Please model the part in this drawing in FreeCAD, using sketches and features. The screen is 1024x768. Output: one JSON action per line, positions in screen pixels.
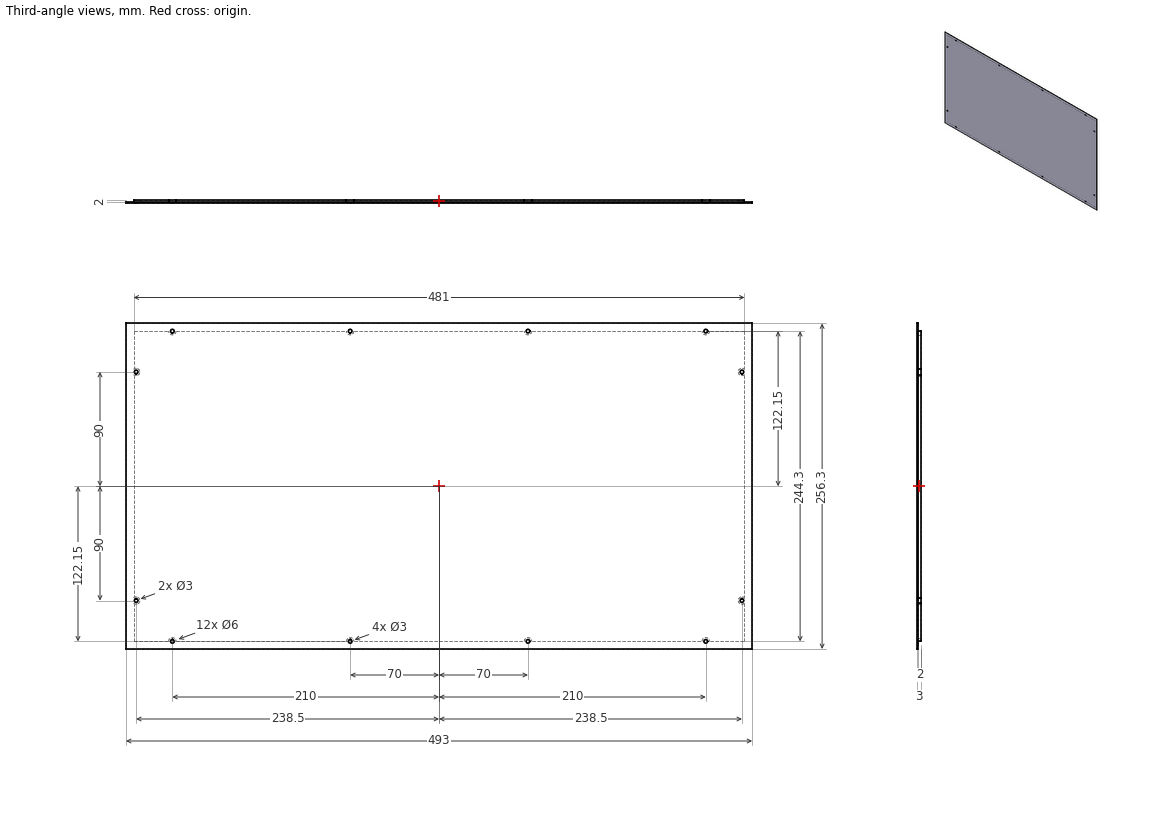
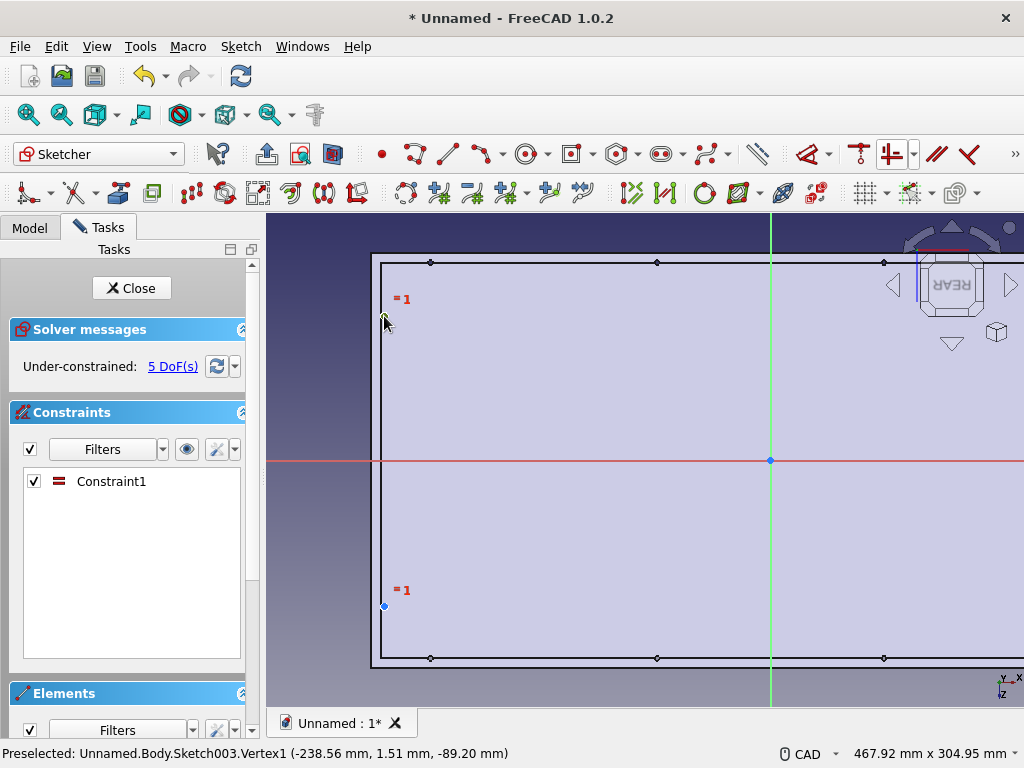
{"action": "left_click", "coordinate": [384, 607]}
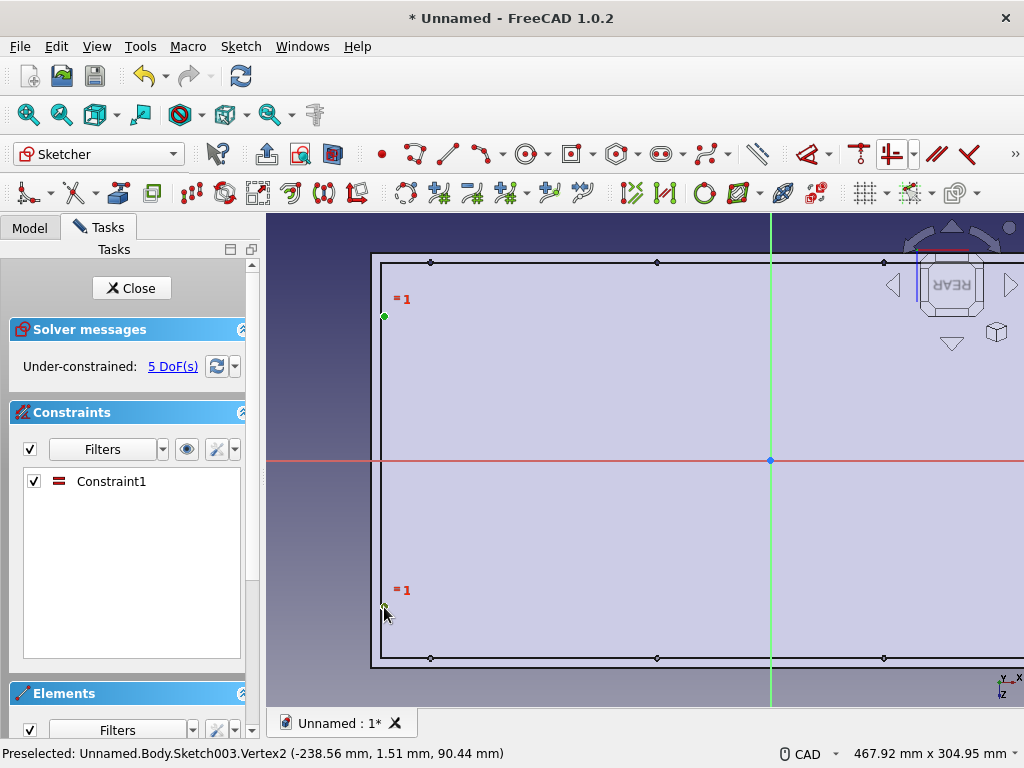
{"action": "key", "text": "v"}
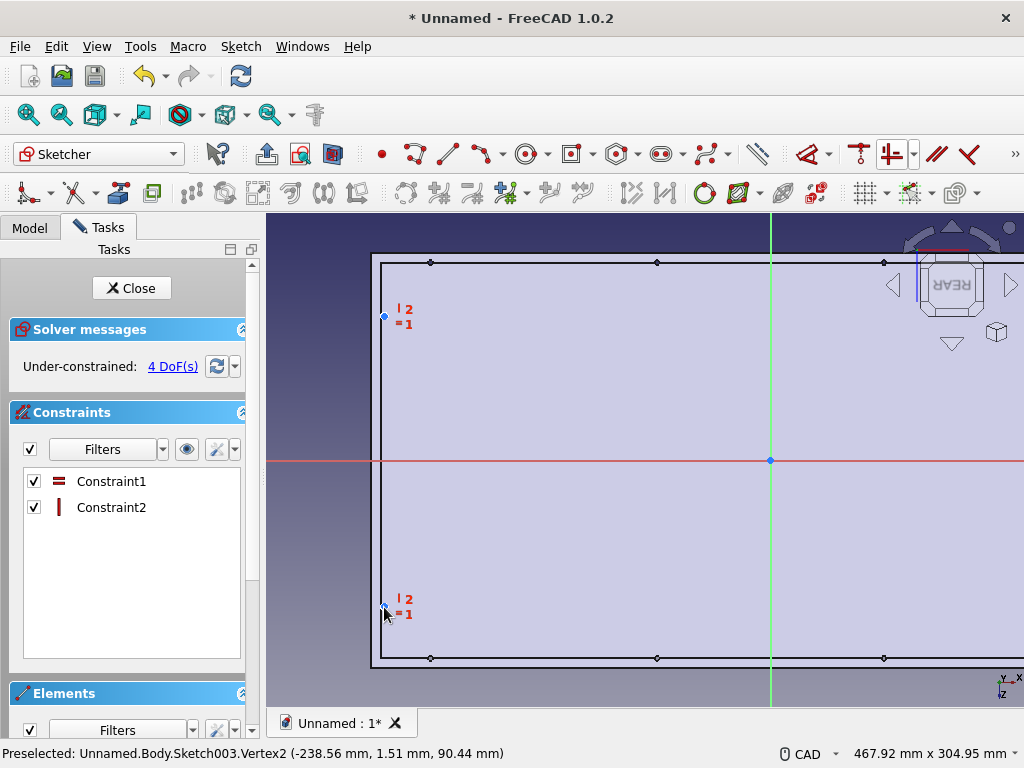
{"action": "left_click", "coordinate": [806, 154]}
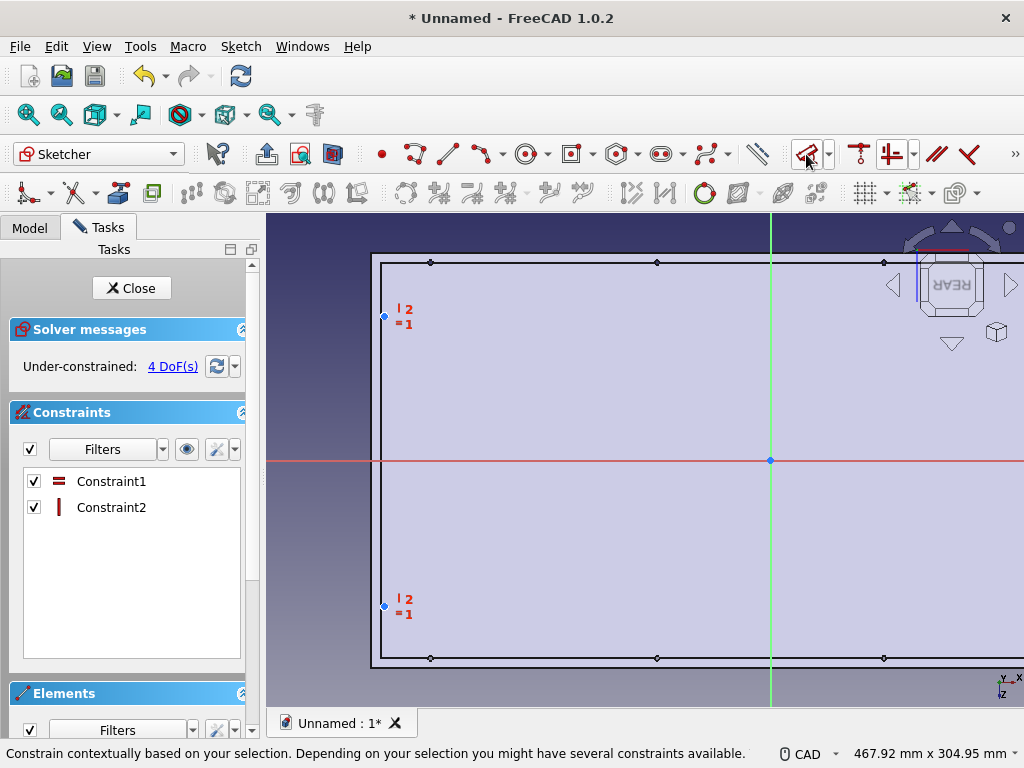
{"action": "scroll", "coordinate": [381, 316], "scroll_direction": "up", "scroll_amount": 11}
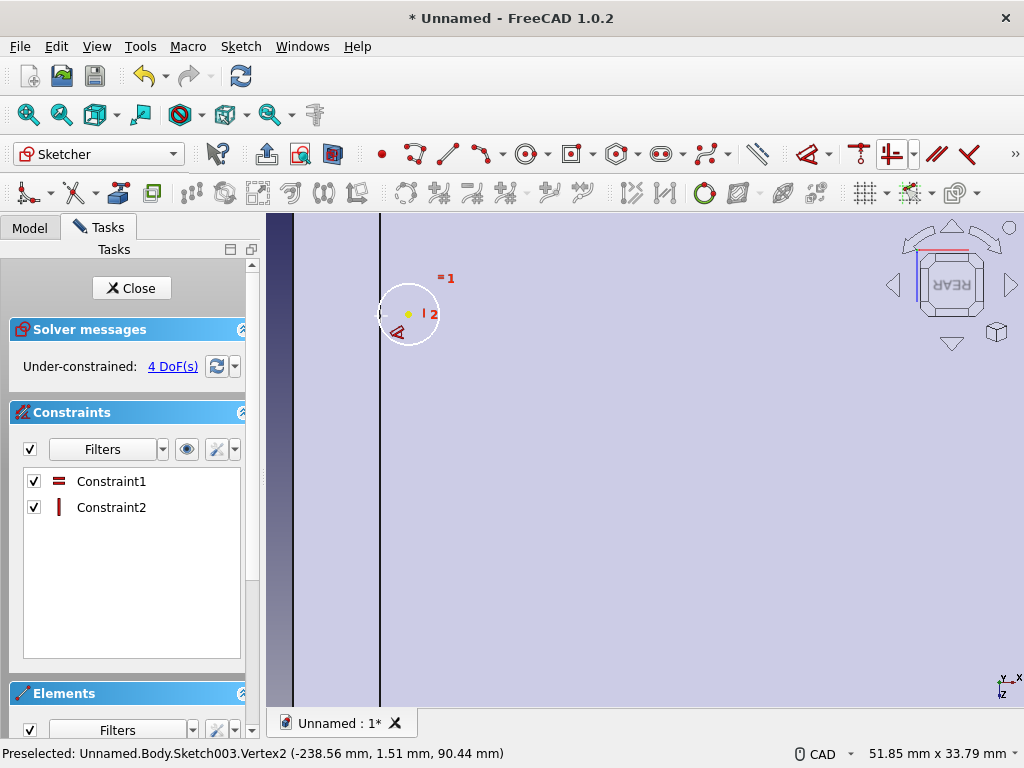
{"action": "left_click", "coordinate": [378, 313]}
{"action": "left_click", "coordinate": [346, 312]}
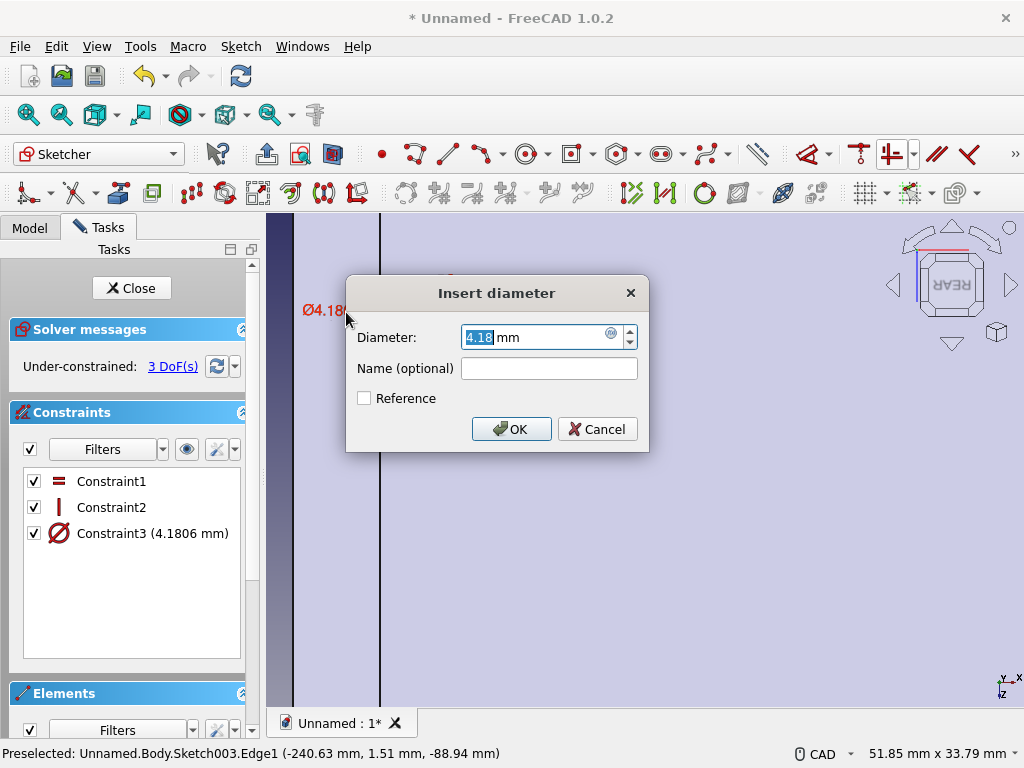
{"action": "type", "text": "3"}
{"action": "key", "text": "Return"}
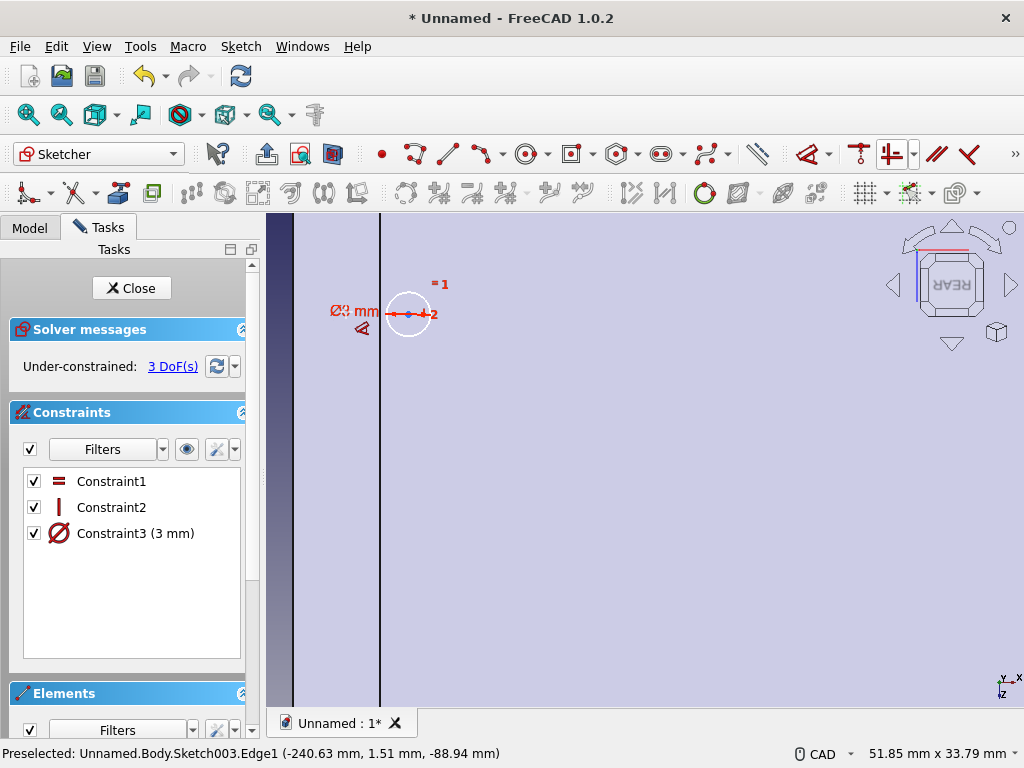
{"action": "scroll", "coordinate": [381, 316], "scroll_direction": "down", "scroll_amount": 11}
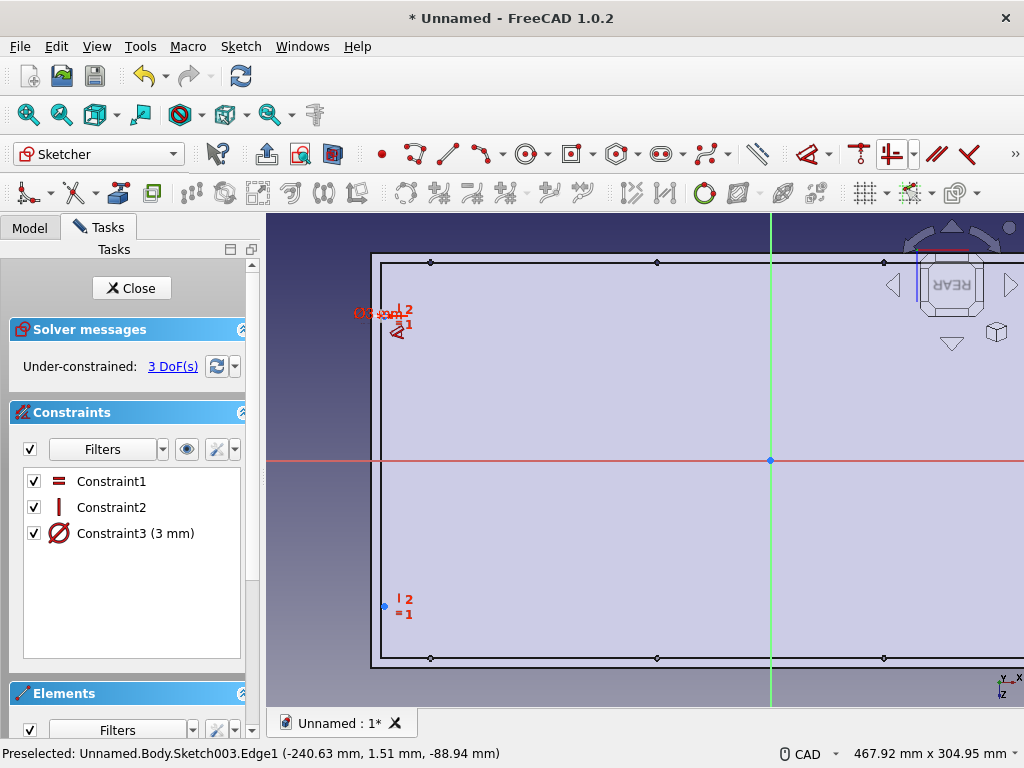
{"action": "left_click", "coordinate": [384, 316]}
{"action": "left_click", "coordinate": [805, 388]}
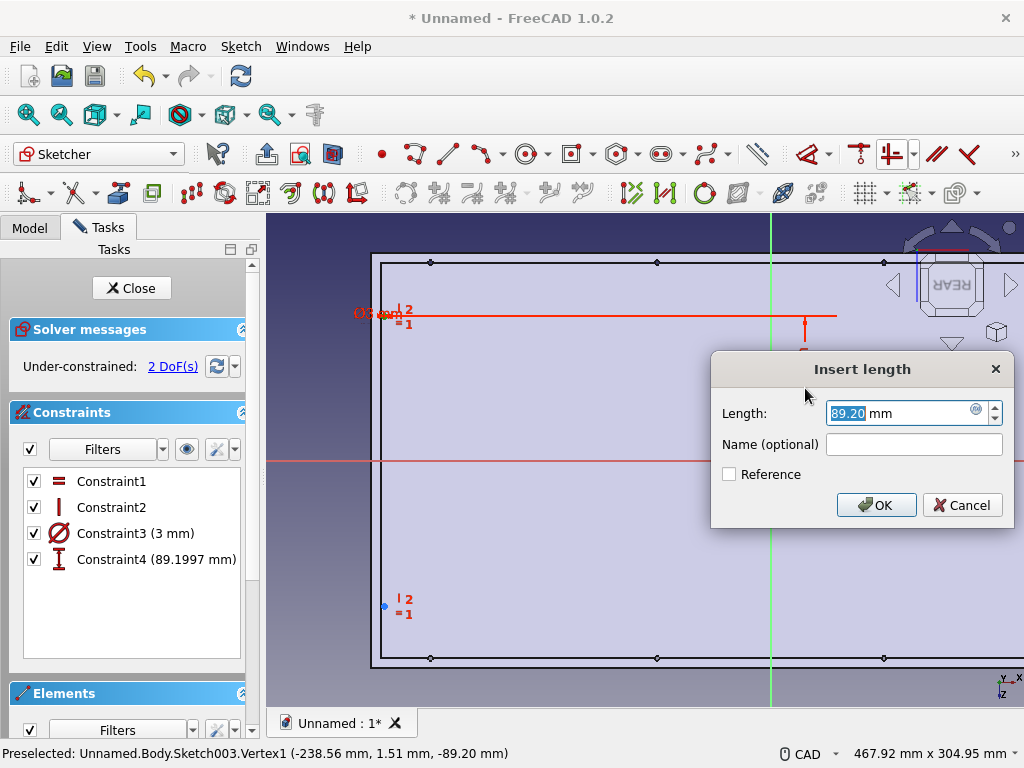
{"action": "type", "text": "90"}
{"action": "key", "text": "Return"}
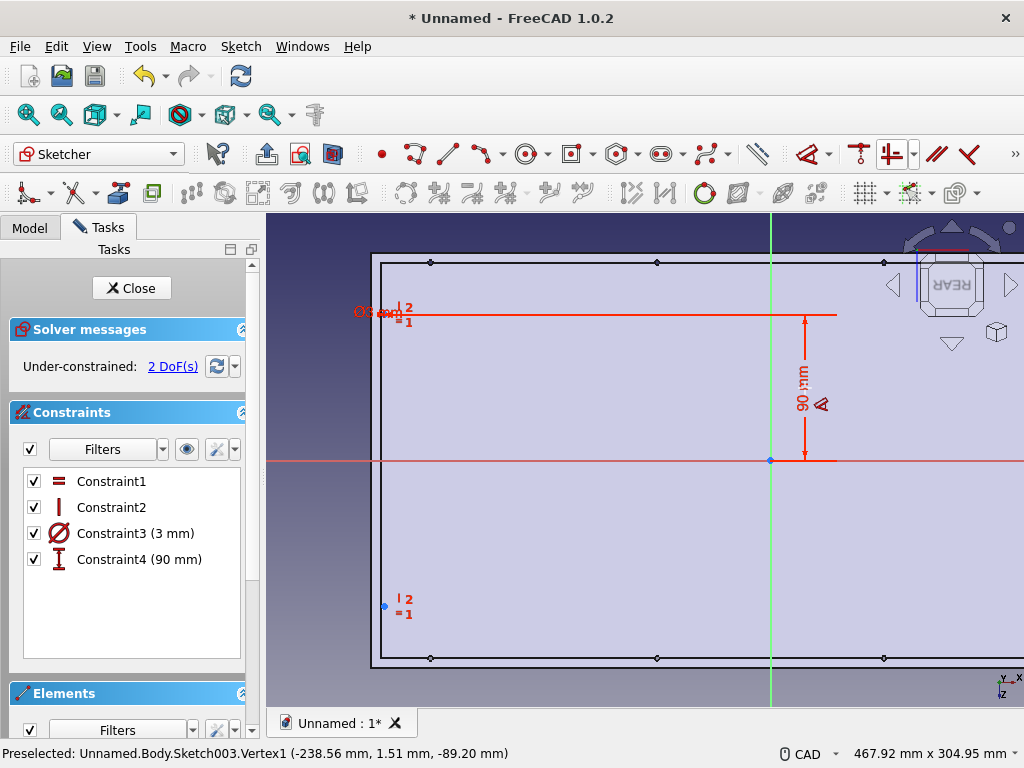
{"action": "left_click", "coordinate": [384, 607]}
{"action": "left_click", "coordinate": [805, 534]}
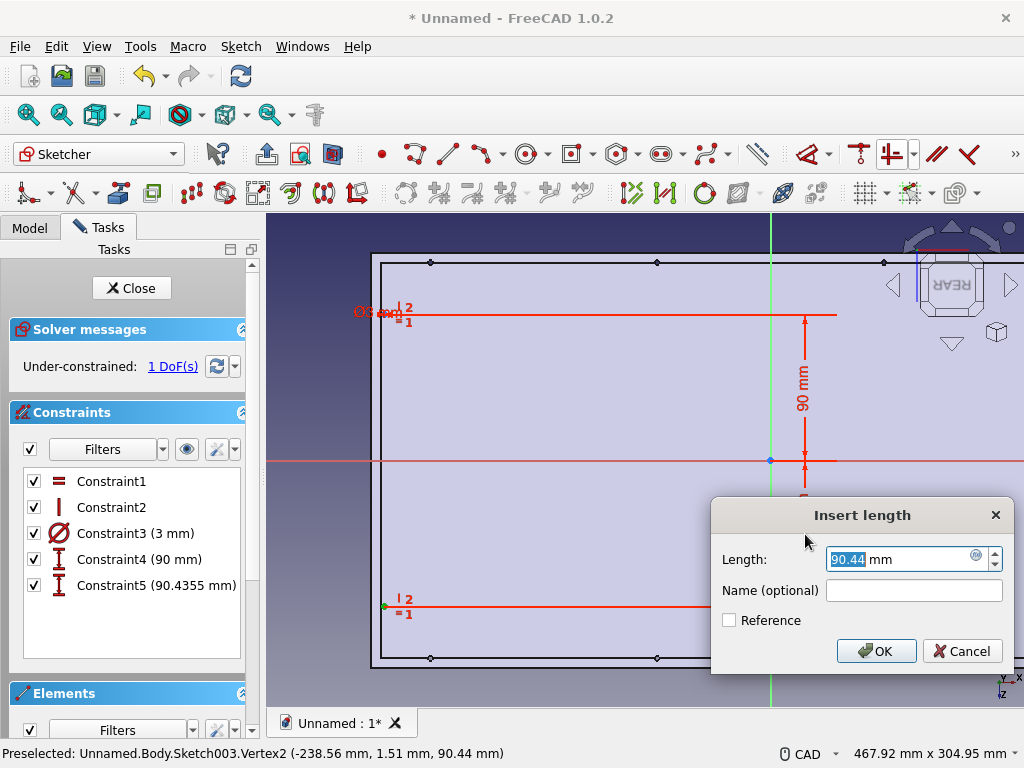
{"action": "type", "text": "90"}
{"action": "key", "text": "Return"}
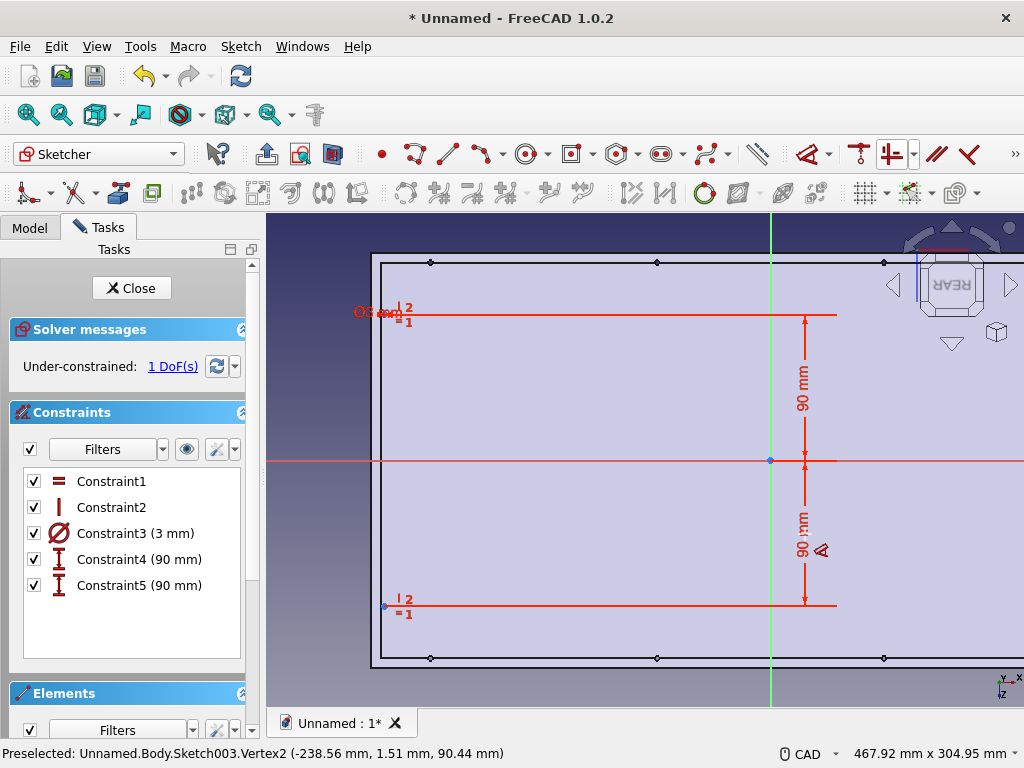
{"action": "left_click", "coordinate": [384, 315]}
{"action": "left_click", "coordinate": [577, 281]}